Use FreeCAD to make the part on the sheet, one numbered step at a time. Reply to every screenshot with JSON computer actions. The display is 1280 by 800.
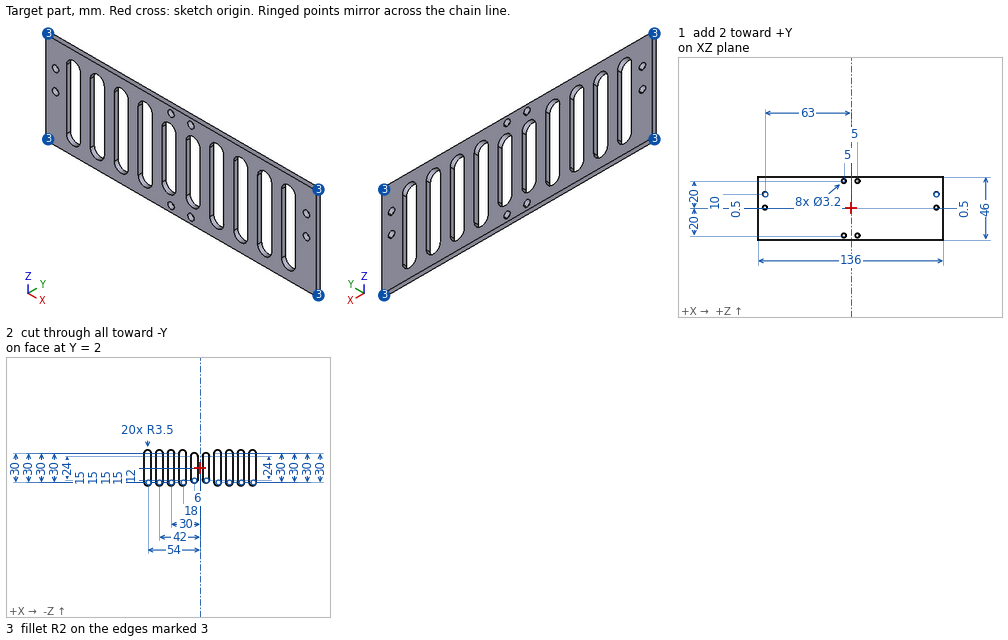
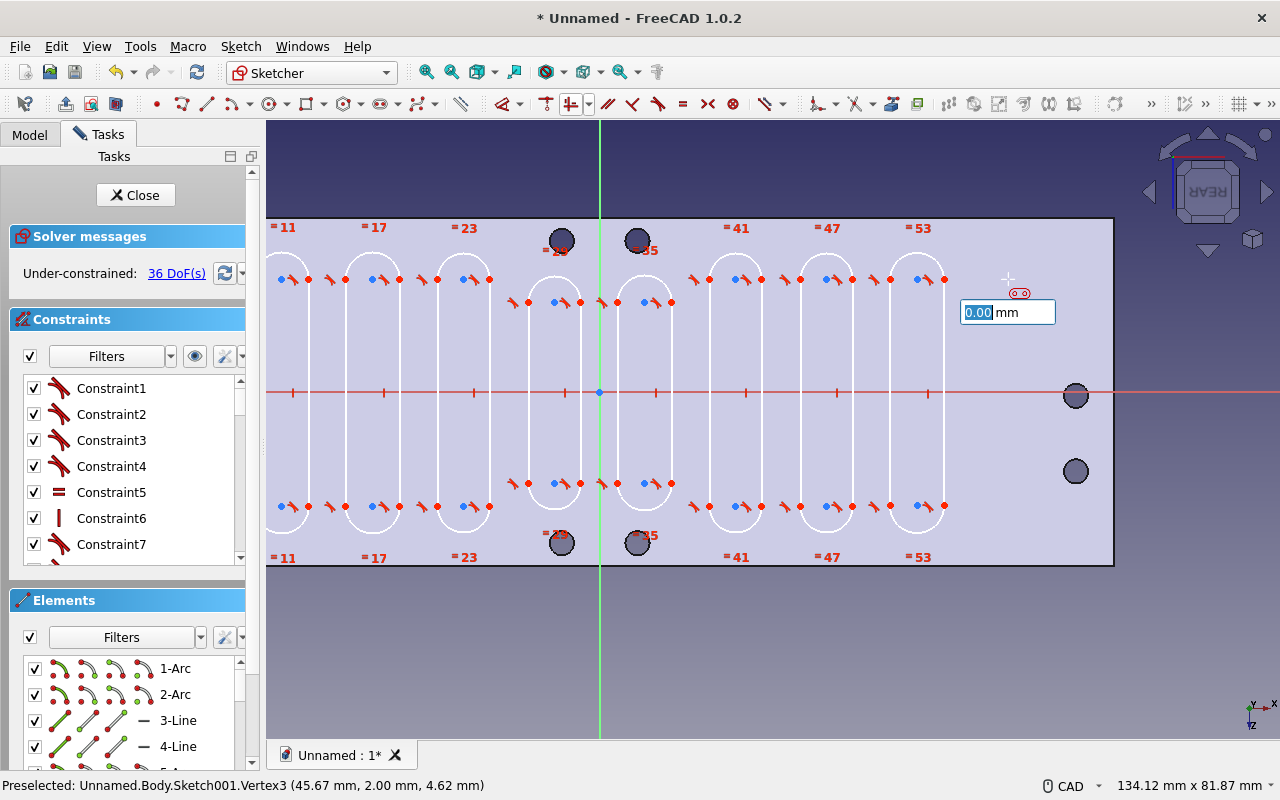
{"action": "left_click", "coordinate": [1034, 426]}
{"action": "key", "text": "Escape"}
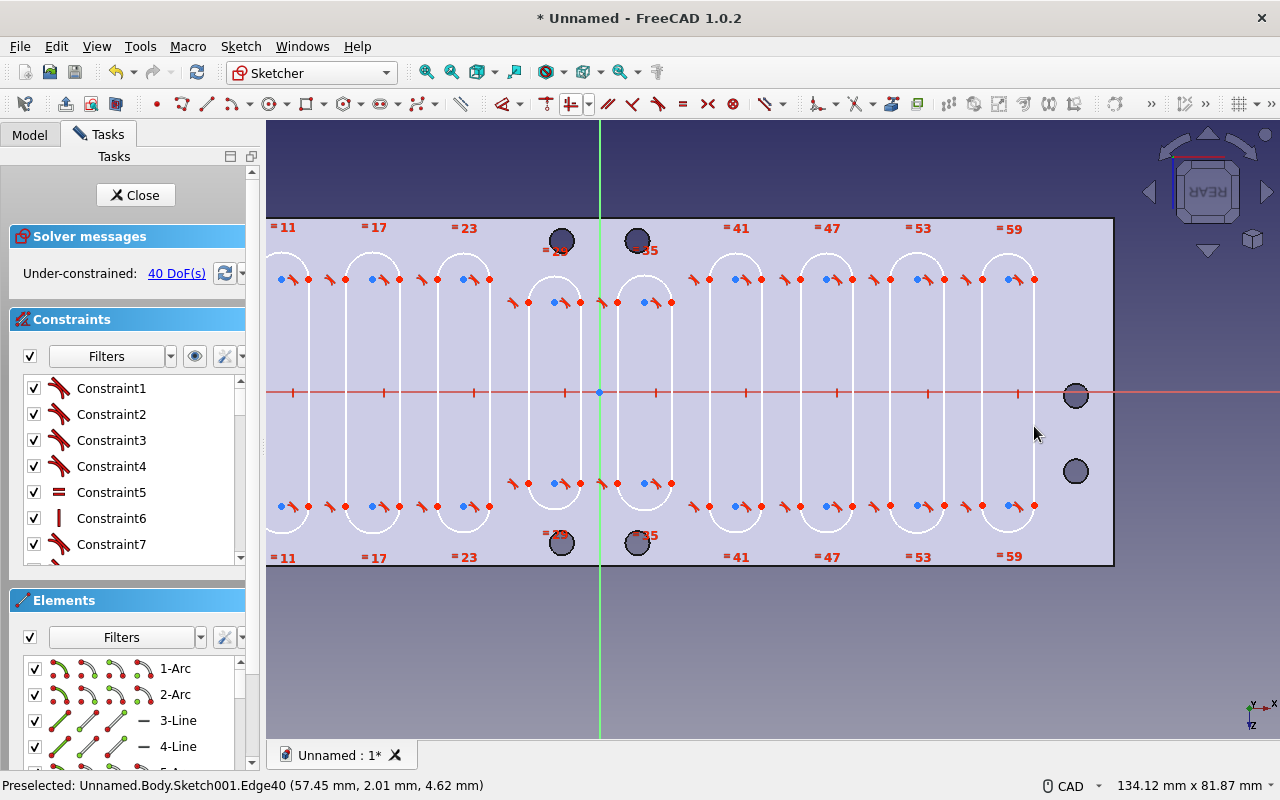
{"action": "scroll", "coordinate": [918, 506], "scroll_direction": "down", "scroll_amount": 2}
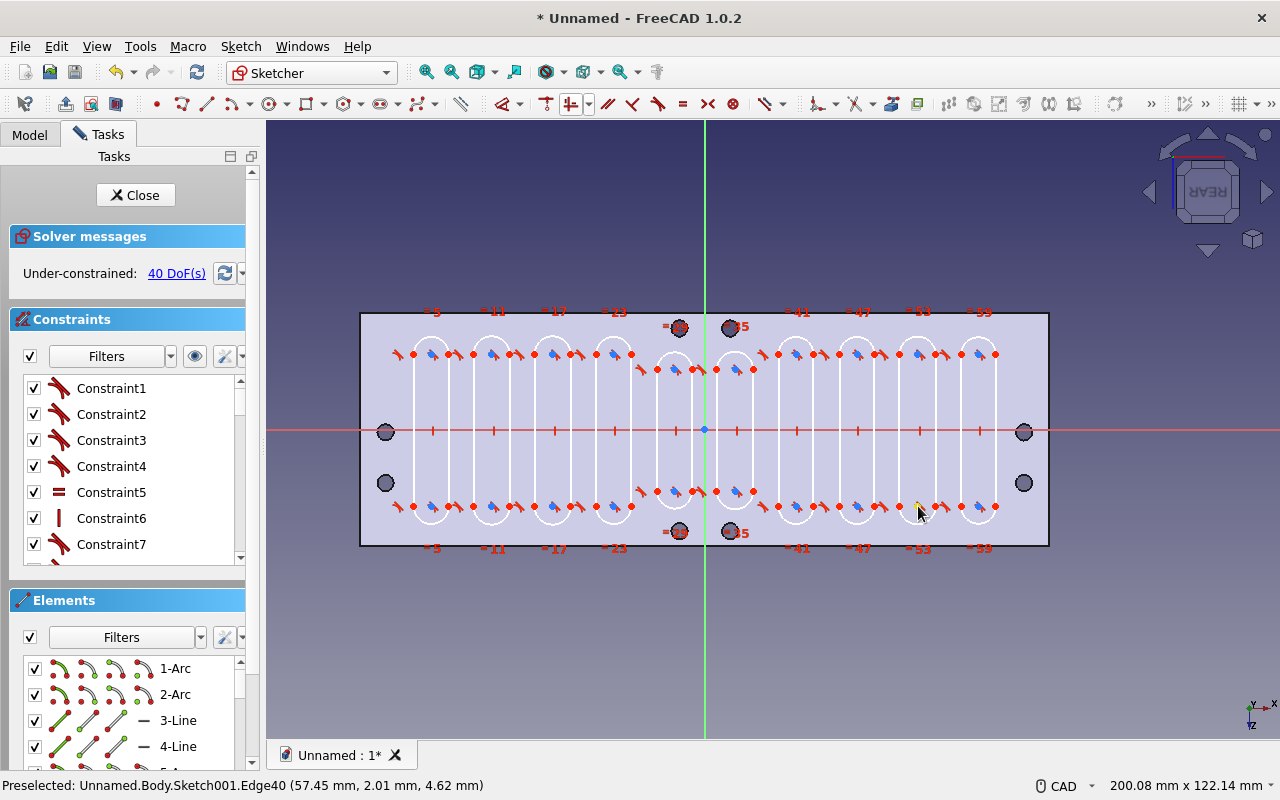
{"action": "left_click", "coordinate": [421, 521]}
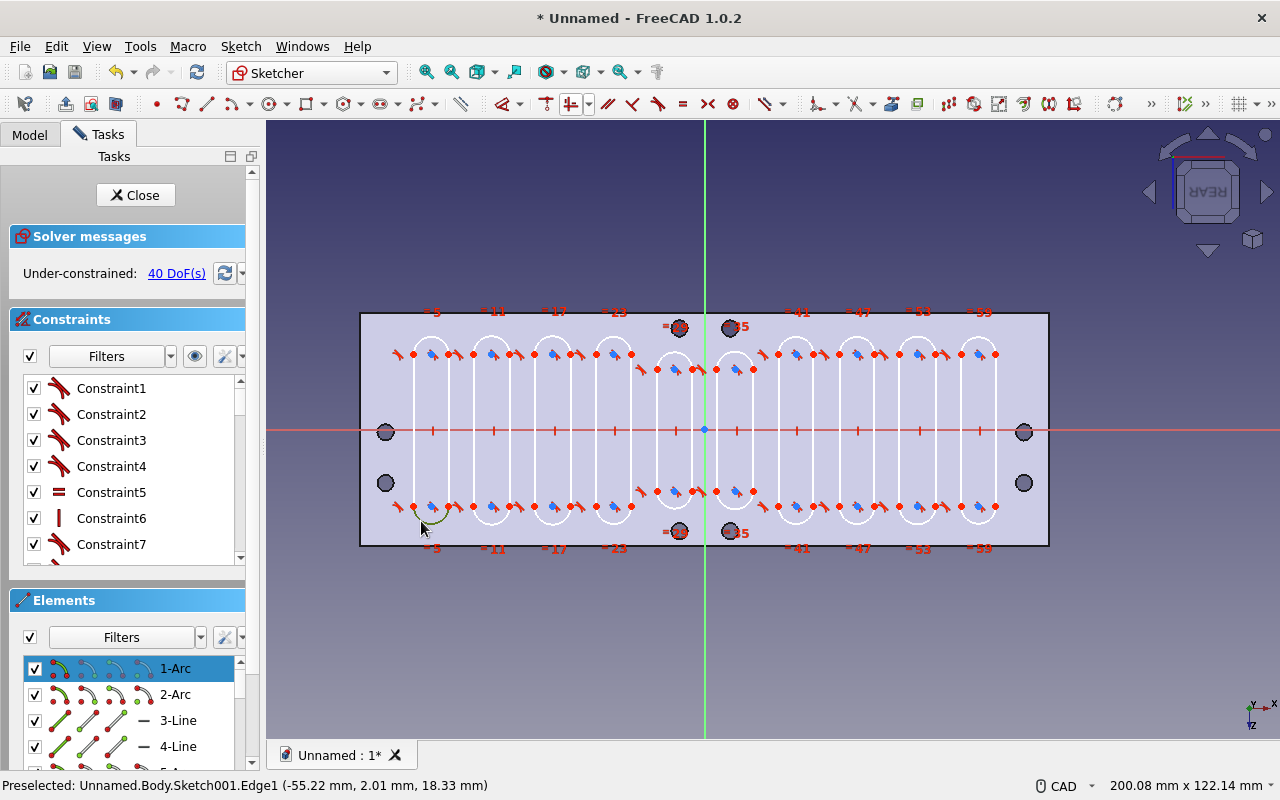
{"action": "left_click", "coordinate": [481, 521]}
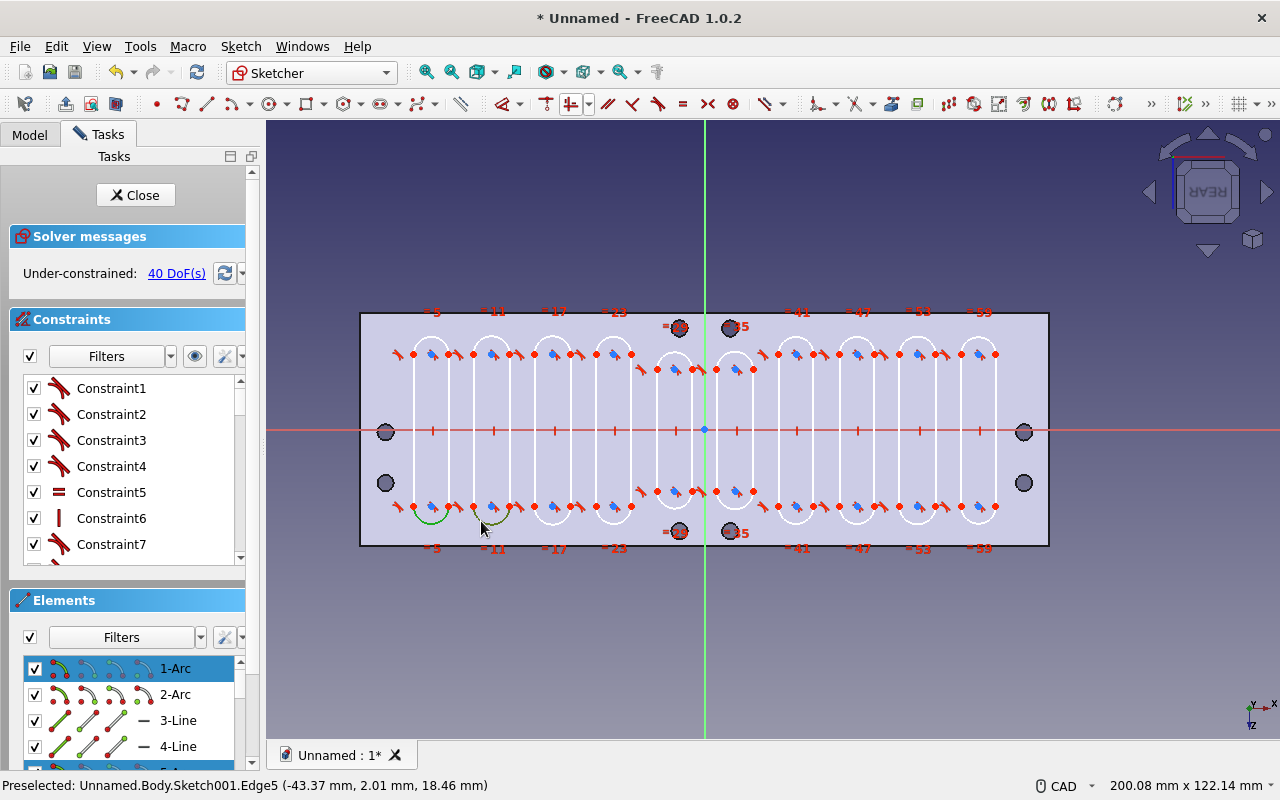
{"action": "left_click", "coordinate": [542, 521]}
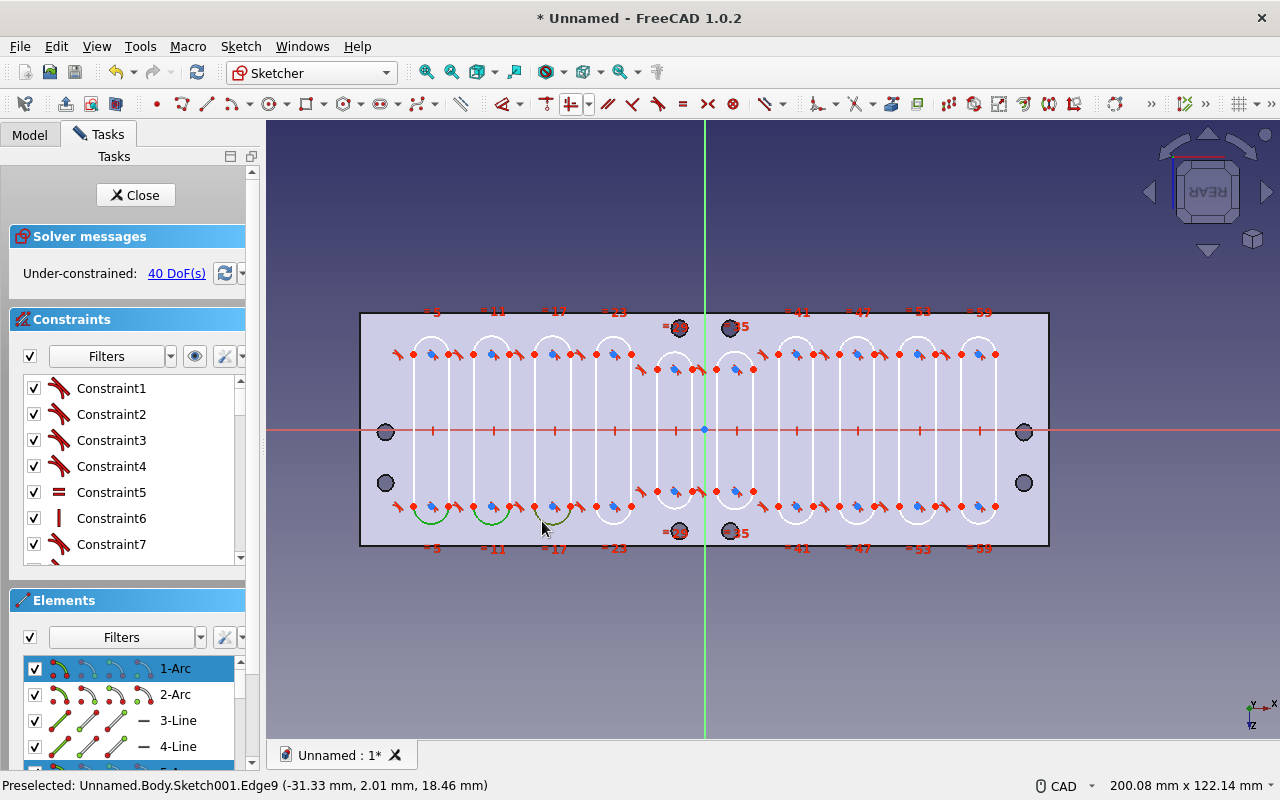
{"action": "left_click", "coordinate": [603, 521]}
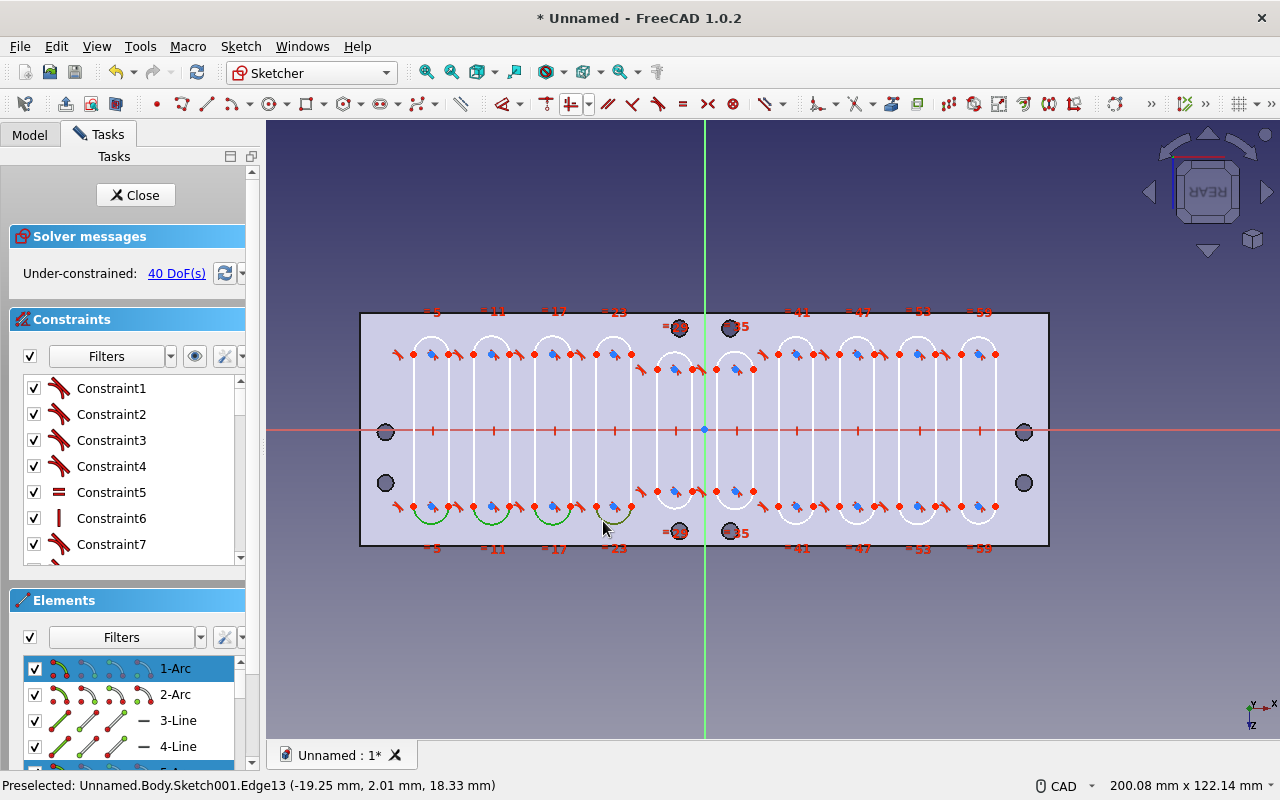
{"action": "left_click", "coordinate": [664, 505]}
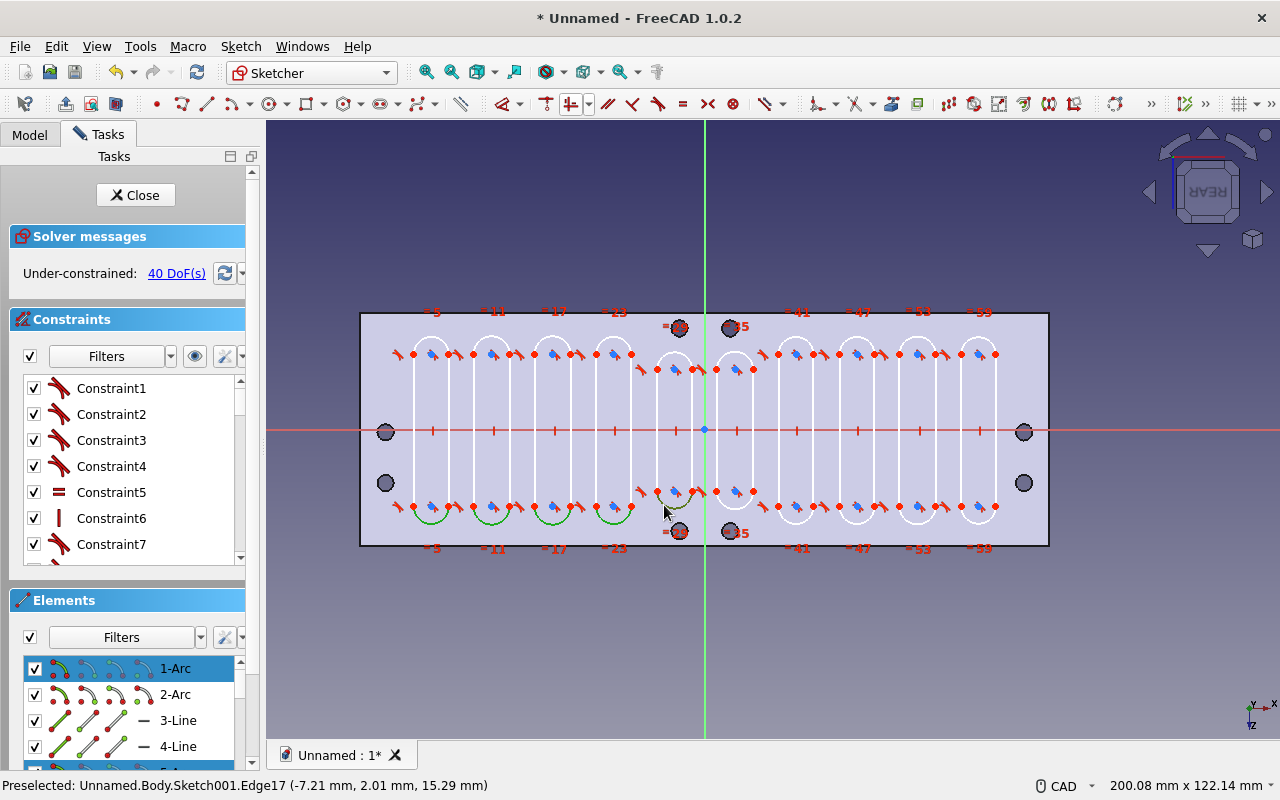
{"action": "left_click", "coordinate": [724, 506]}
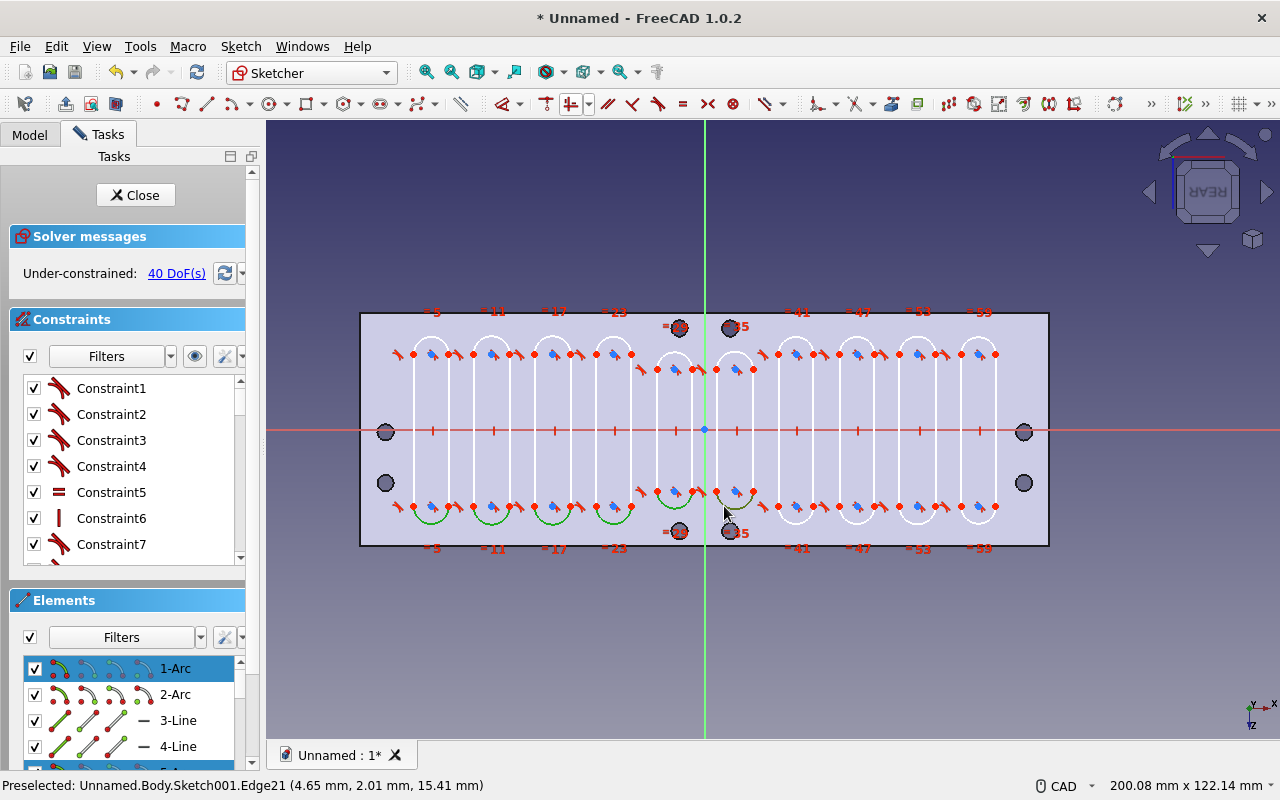
{"action": "left_click", "coordinate": [786, 521]}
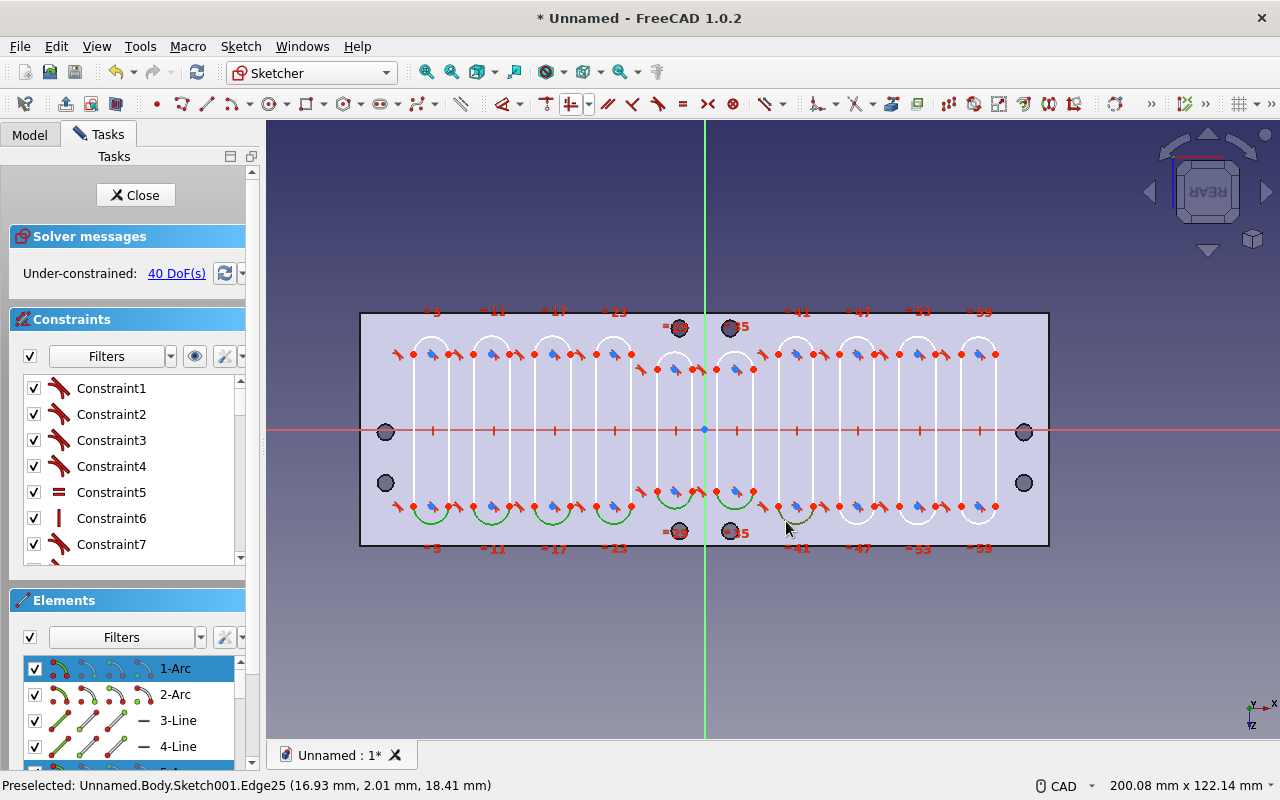
{"action": "left_click", "coordinate": [847, 521]}